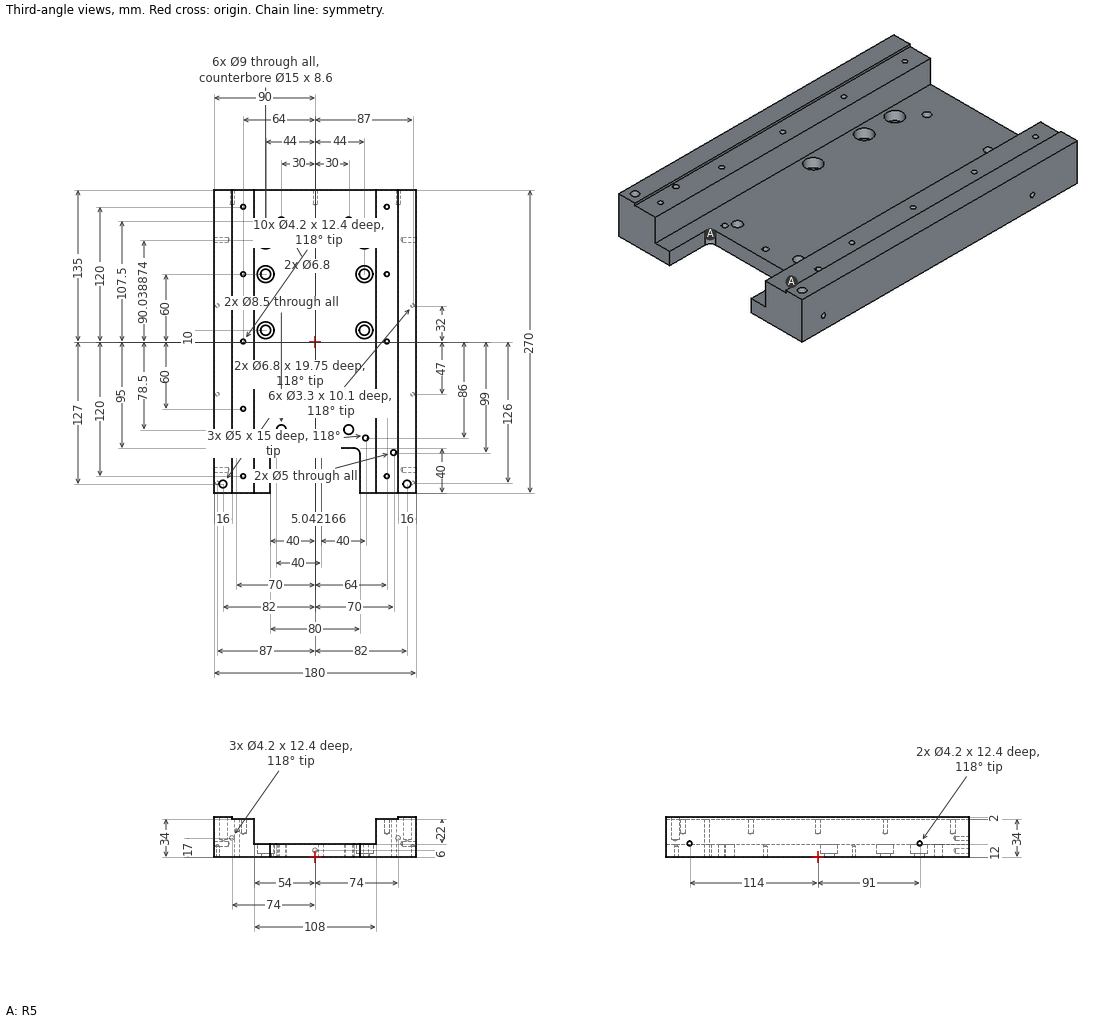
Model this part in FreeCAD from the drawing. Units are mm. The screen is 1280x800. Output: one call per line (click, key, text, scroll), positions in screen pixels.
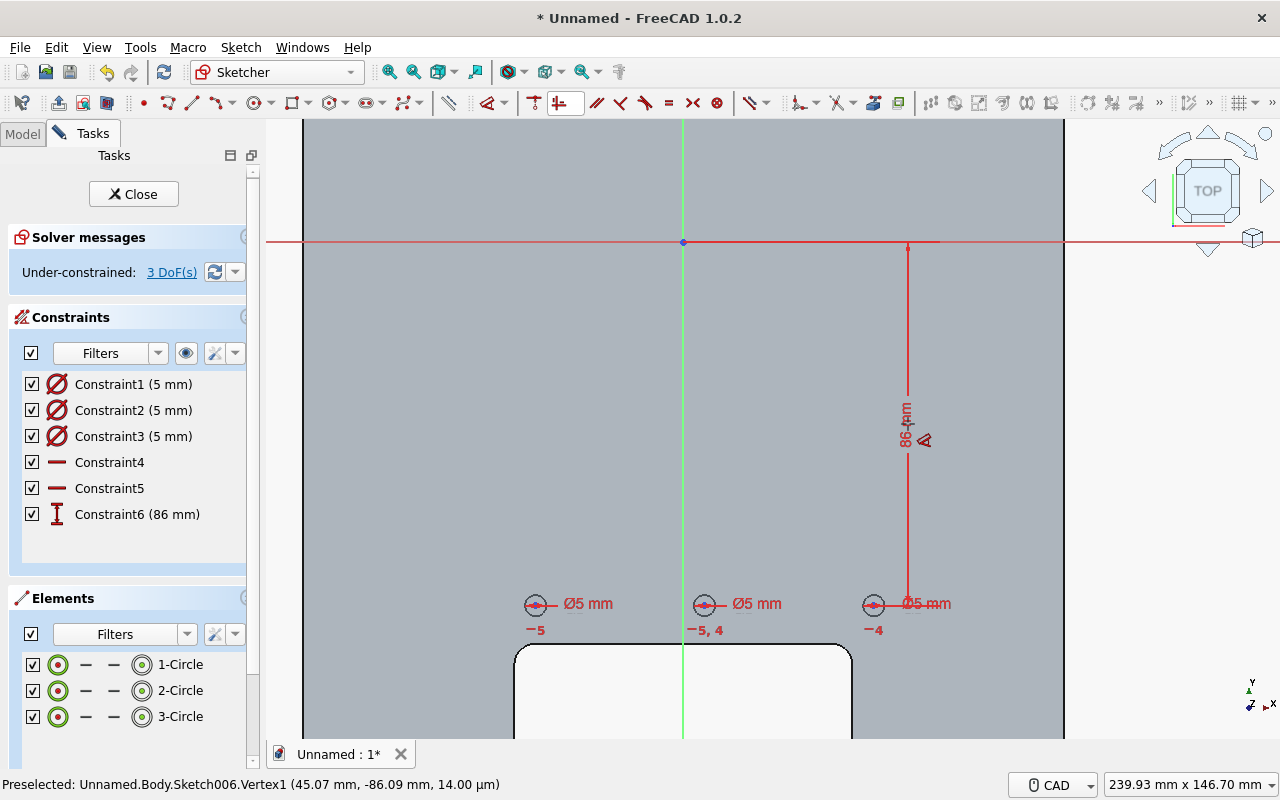
click(874, 606)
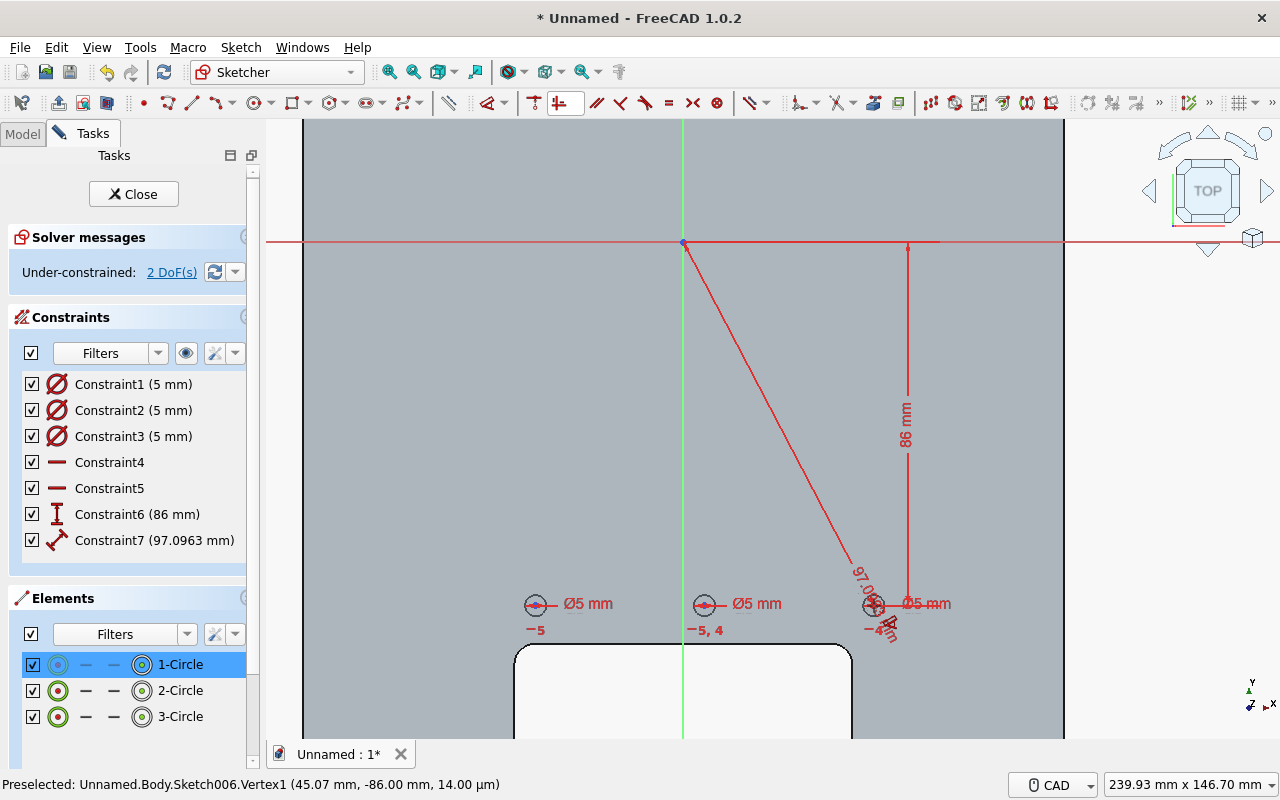
click(704, 606)
click(789, 640)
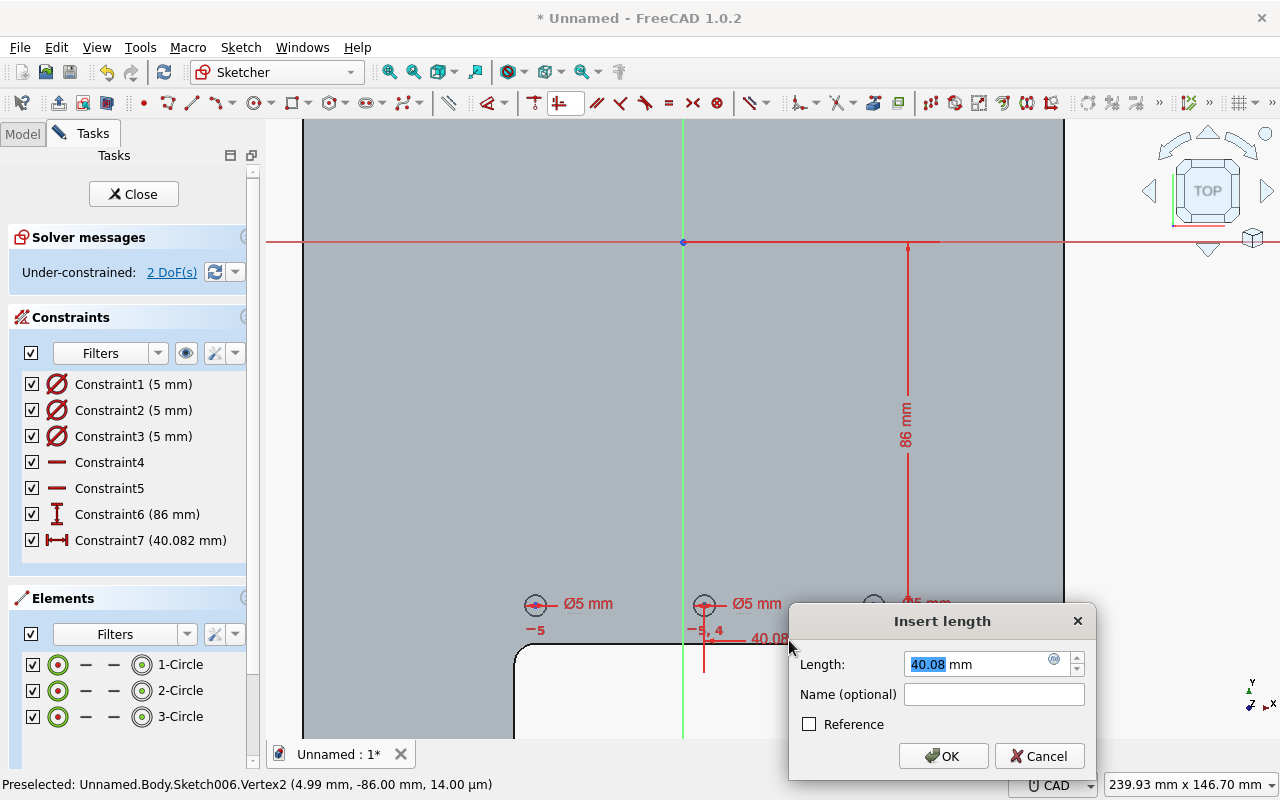
text(40)
key(Return)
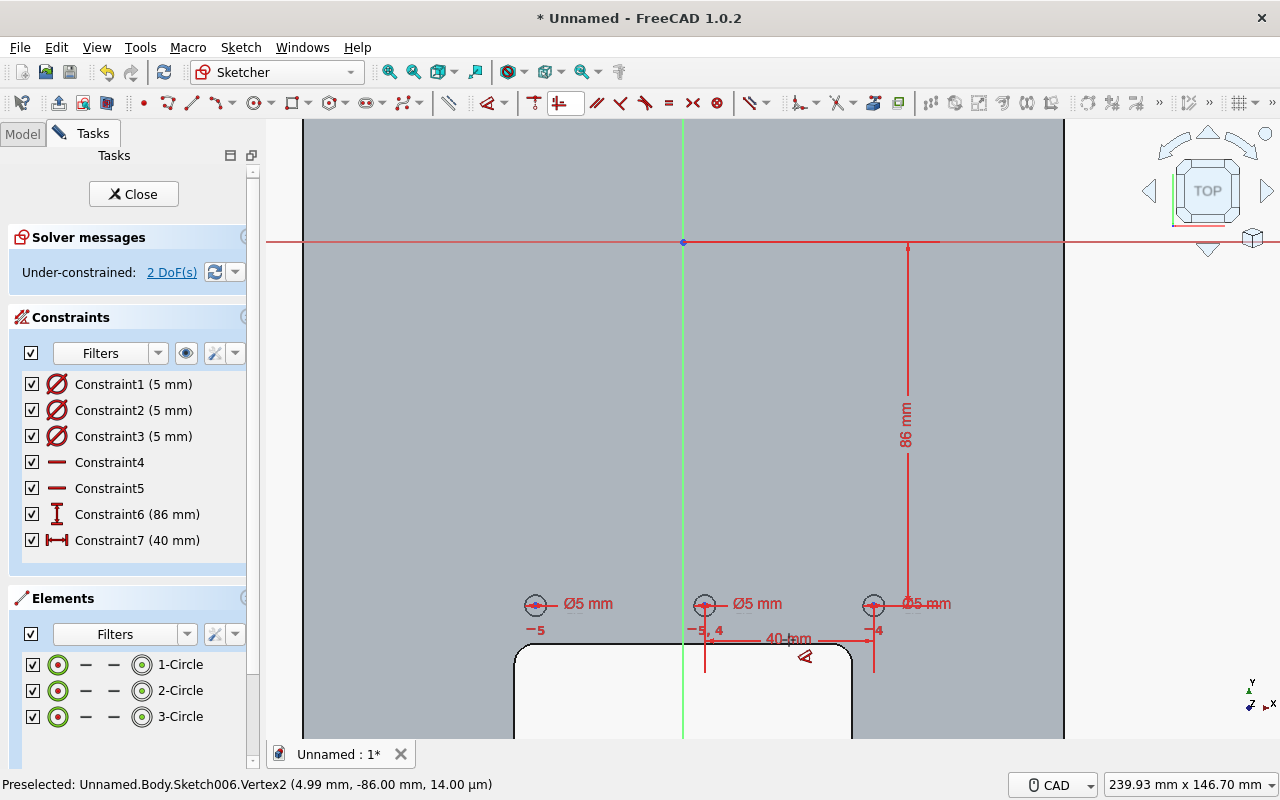
click(705, 606)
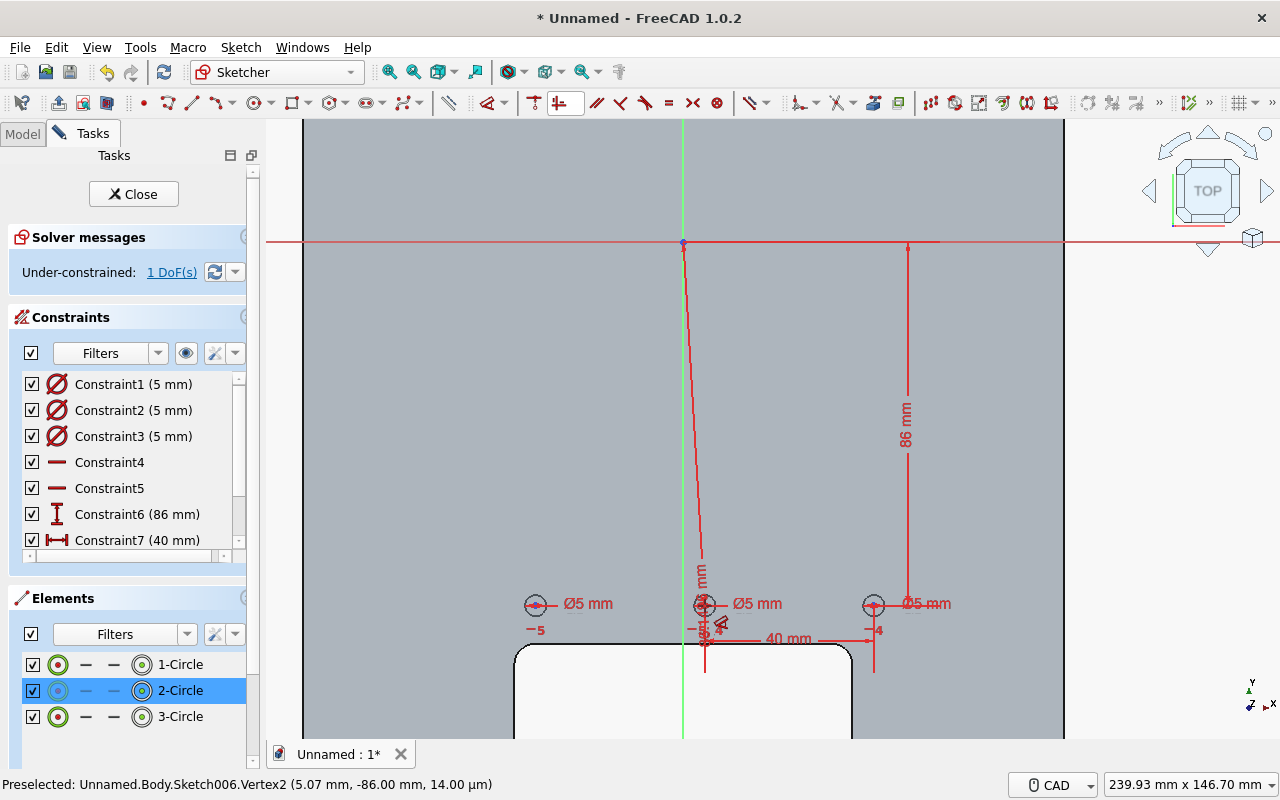
click(536, 606)
click(620, 640)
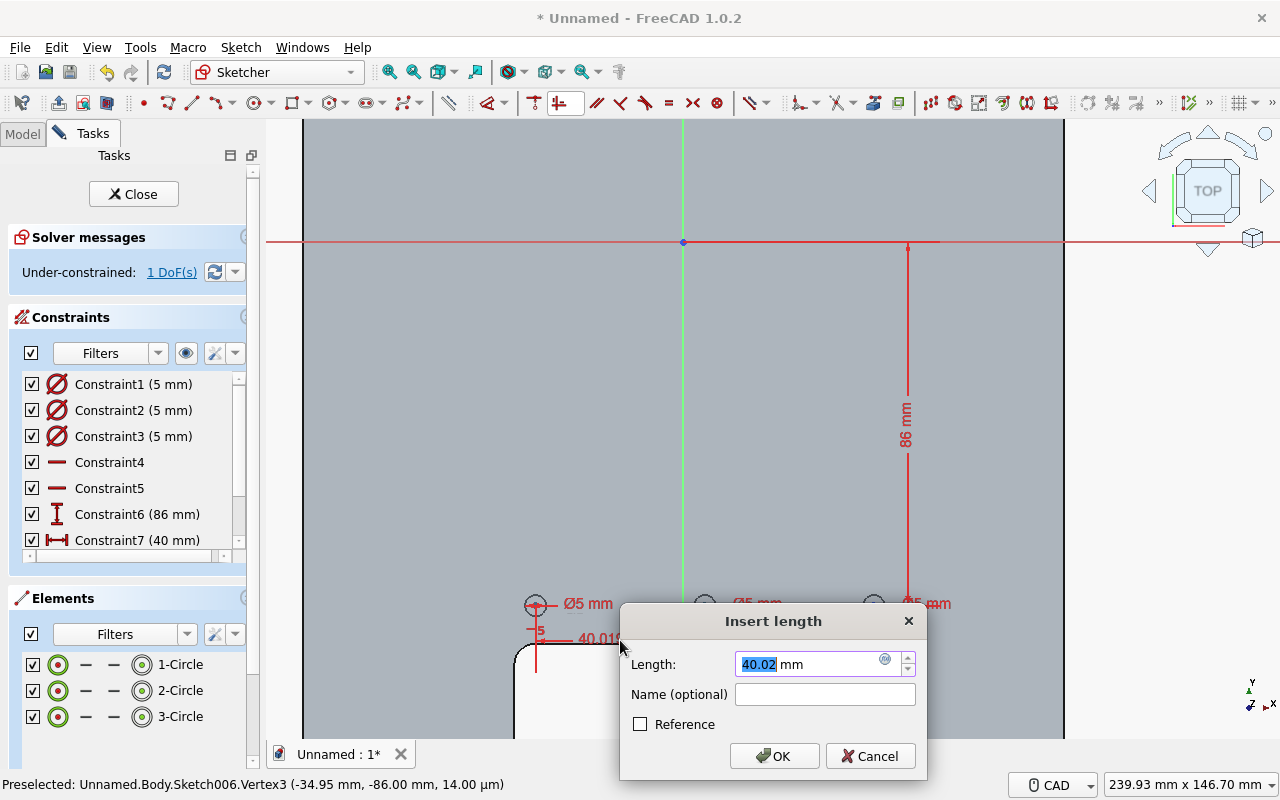
text(40)
key(Return)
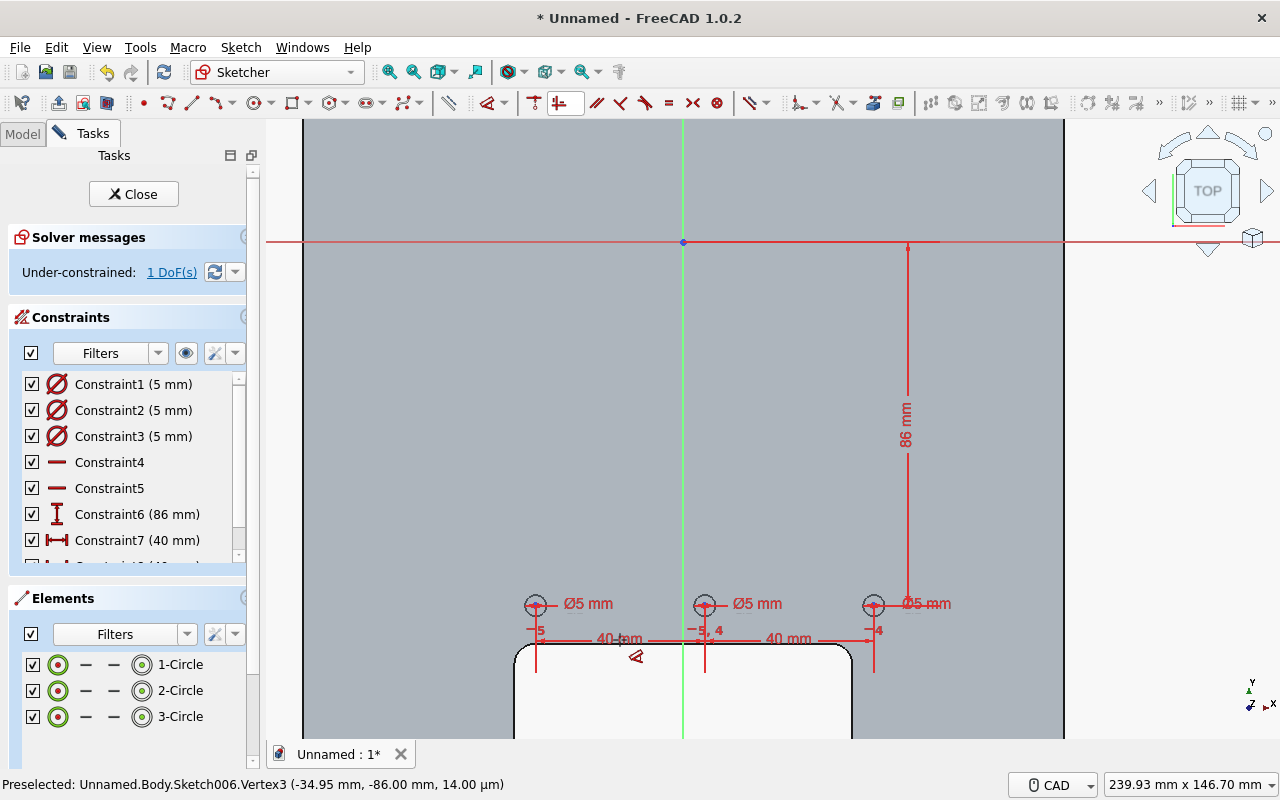
scroll(705, 606, up, 4)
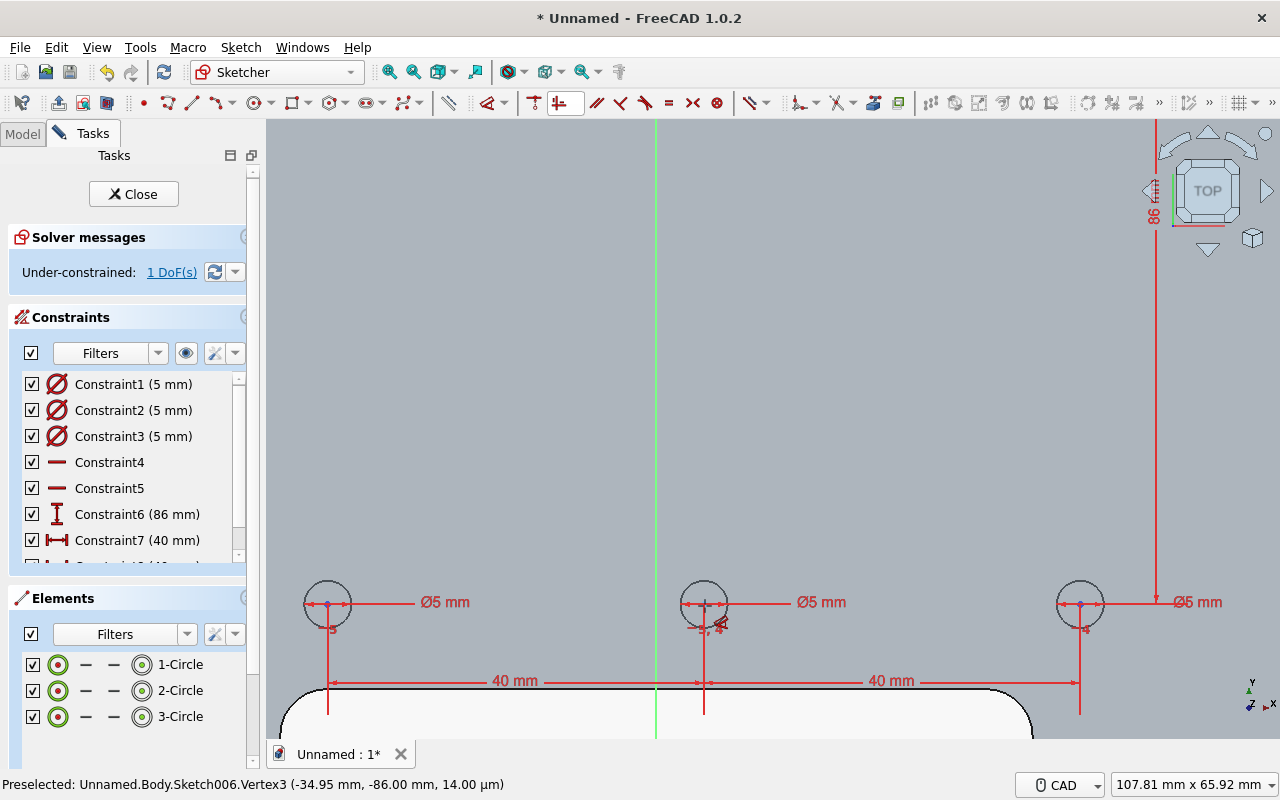
click(704, 604)
click(680, 638)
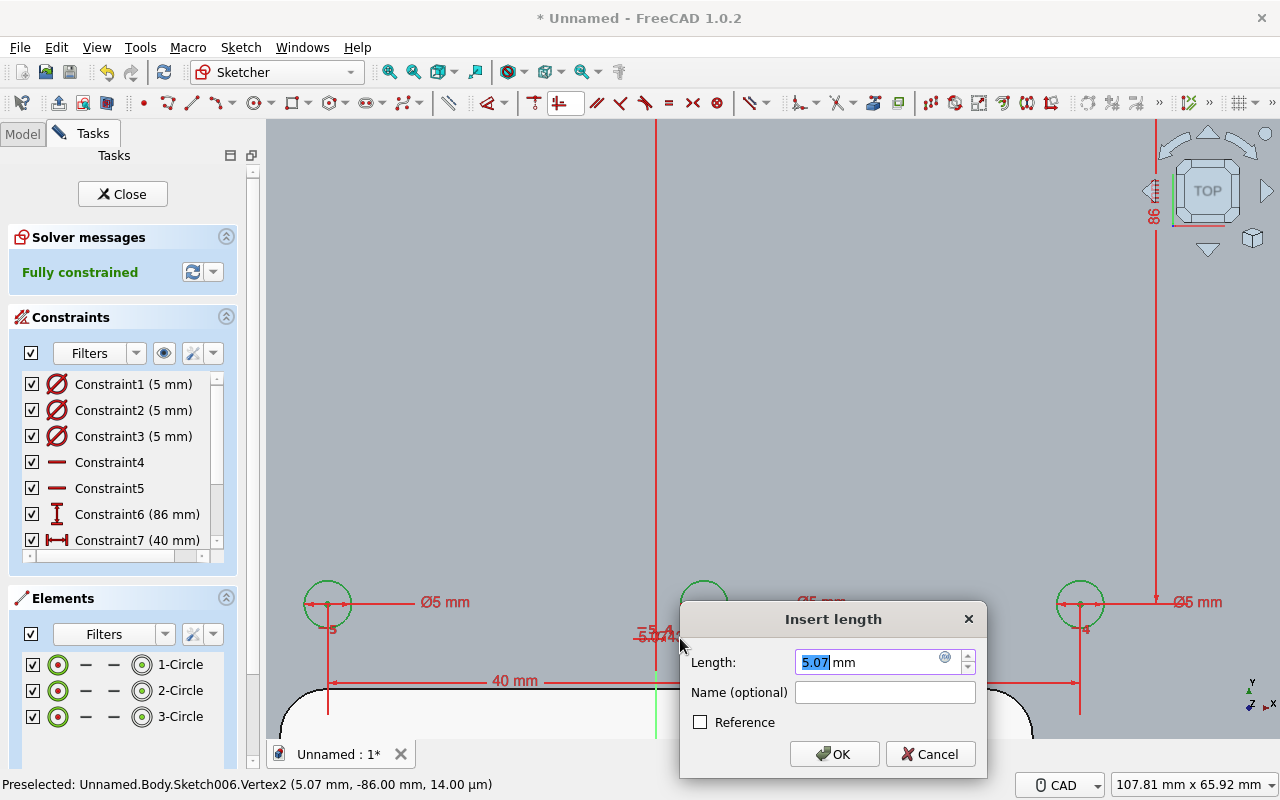
text(5.042166)
key(Return)
key(Escape)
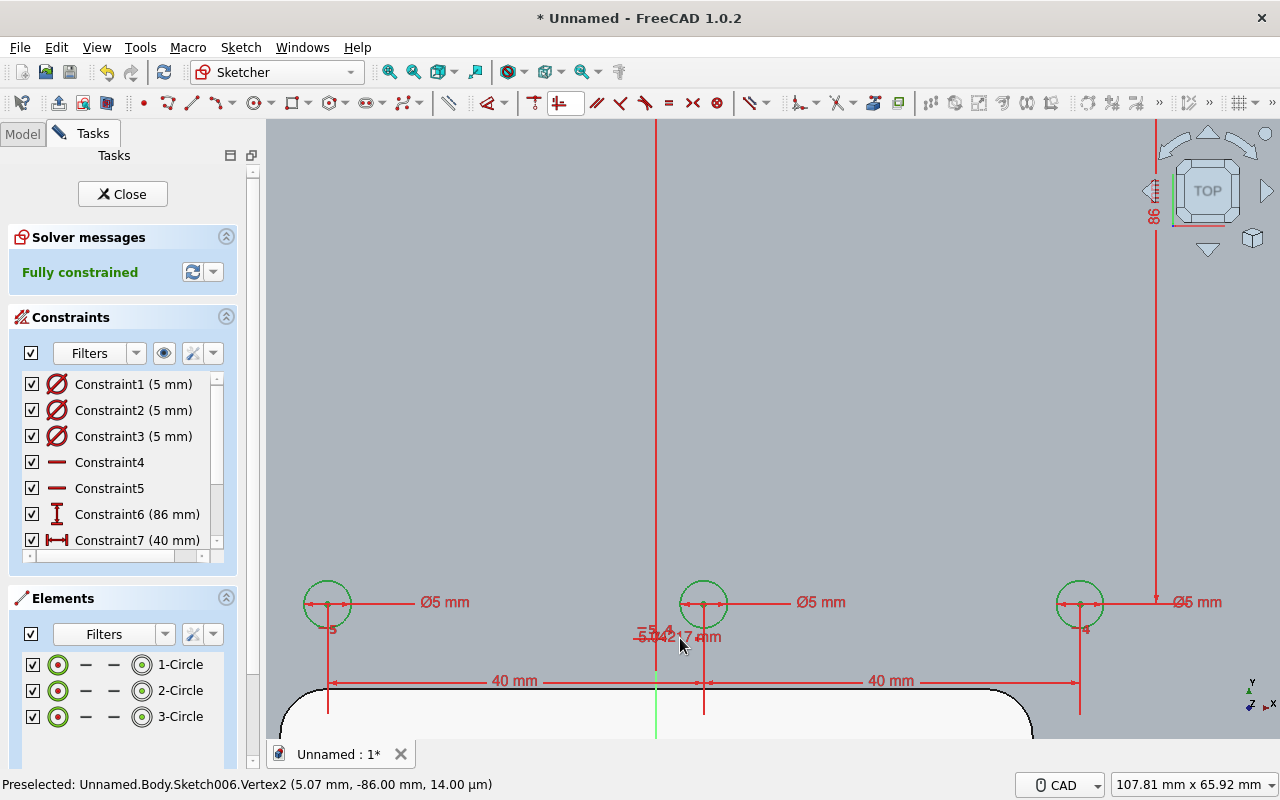
click(123, 194)